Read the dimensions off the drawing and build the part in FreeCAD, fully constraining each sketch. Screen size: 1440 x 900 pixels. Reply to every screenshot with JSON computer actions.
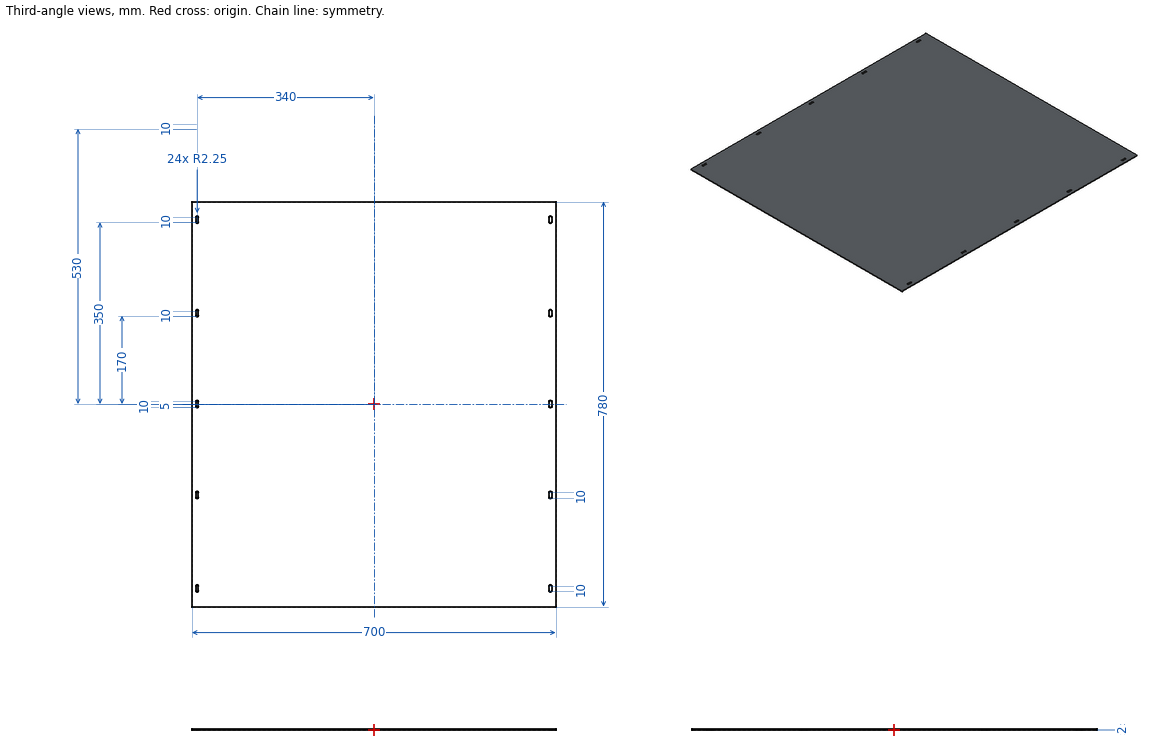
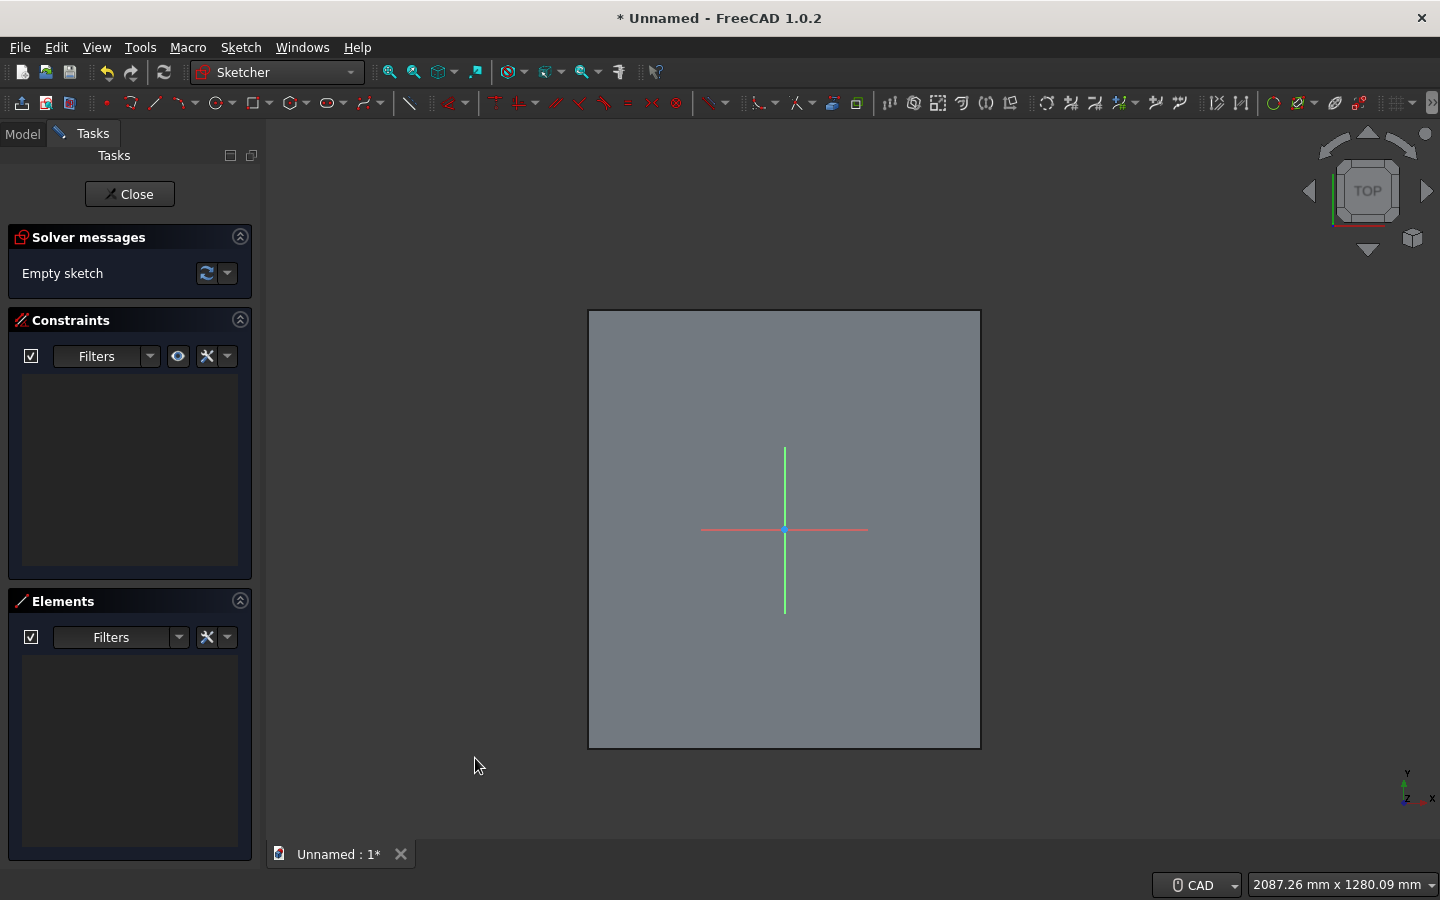
{"action": "key", "text": "g s"}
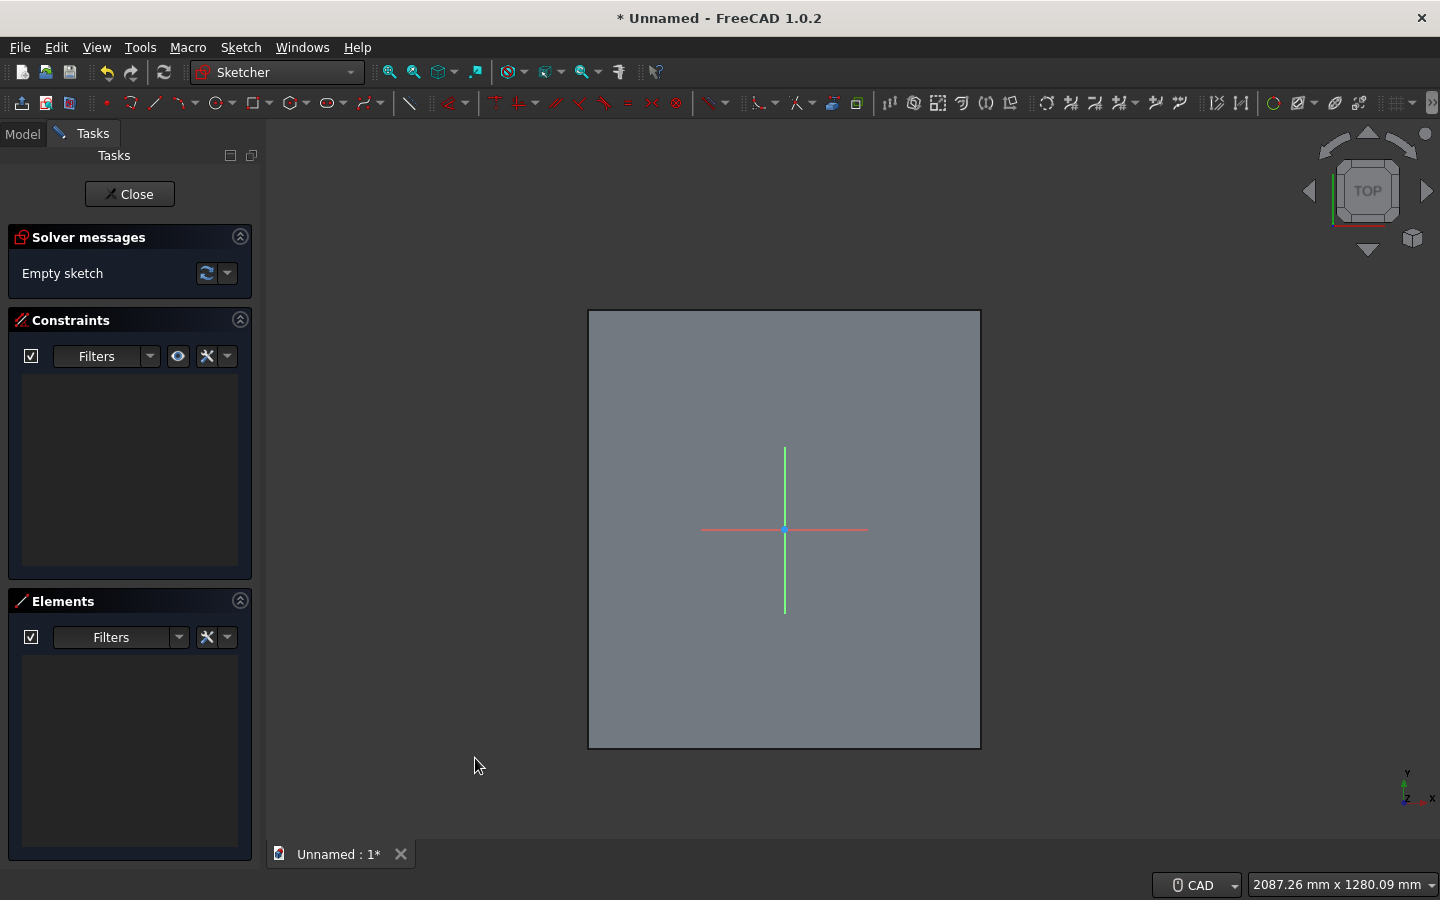
{"action": "scroll", "coordinate": [593, 333], "scroll_direction": "up", "scroll_amount": 15}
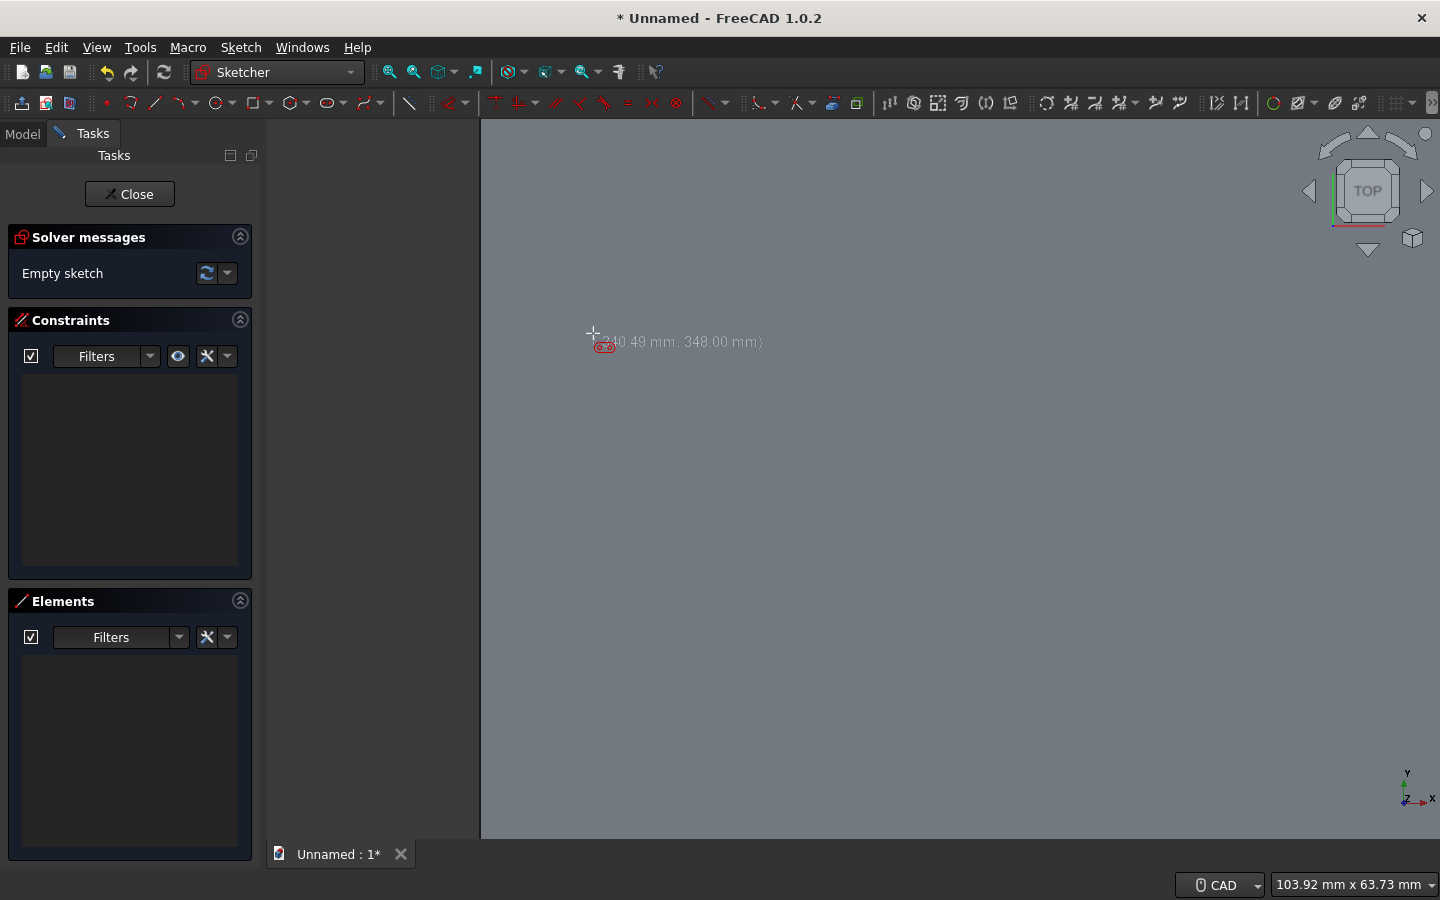
{"action": "scroll", "coordinate": [593, 333], "scroll_direction": "down", "scroll_amount": 15}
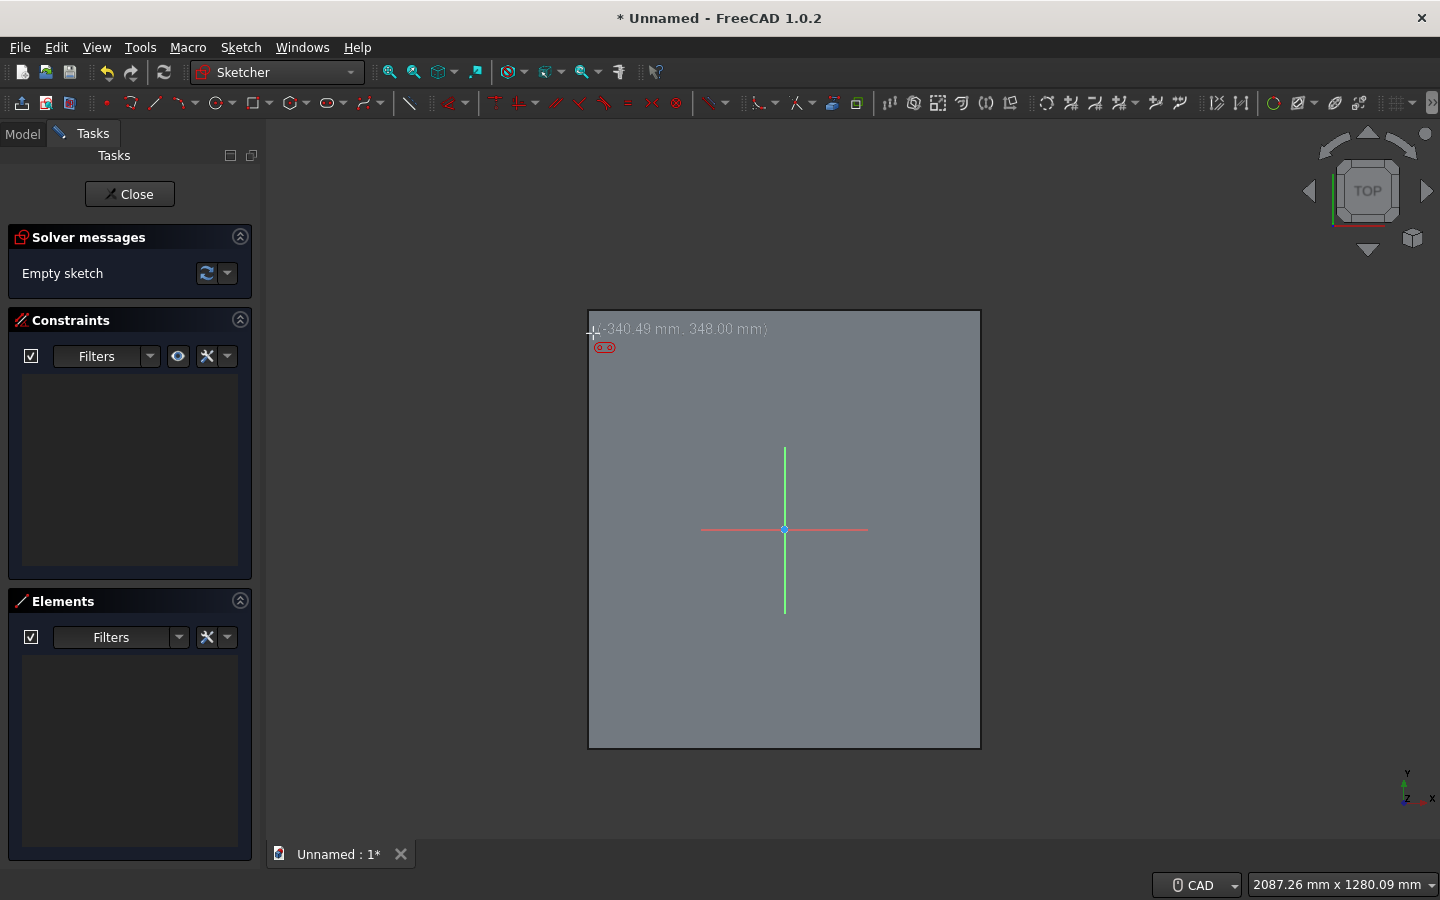
{"action": "left_click", "coordinate": [593, 333]}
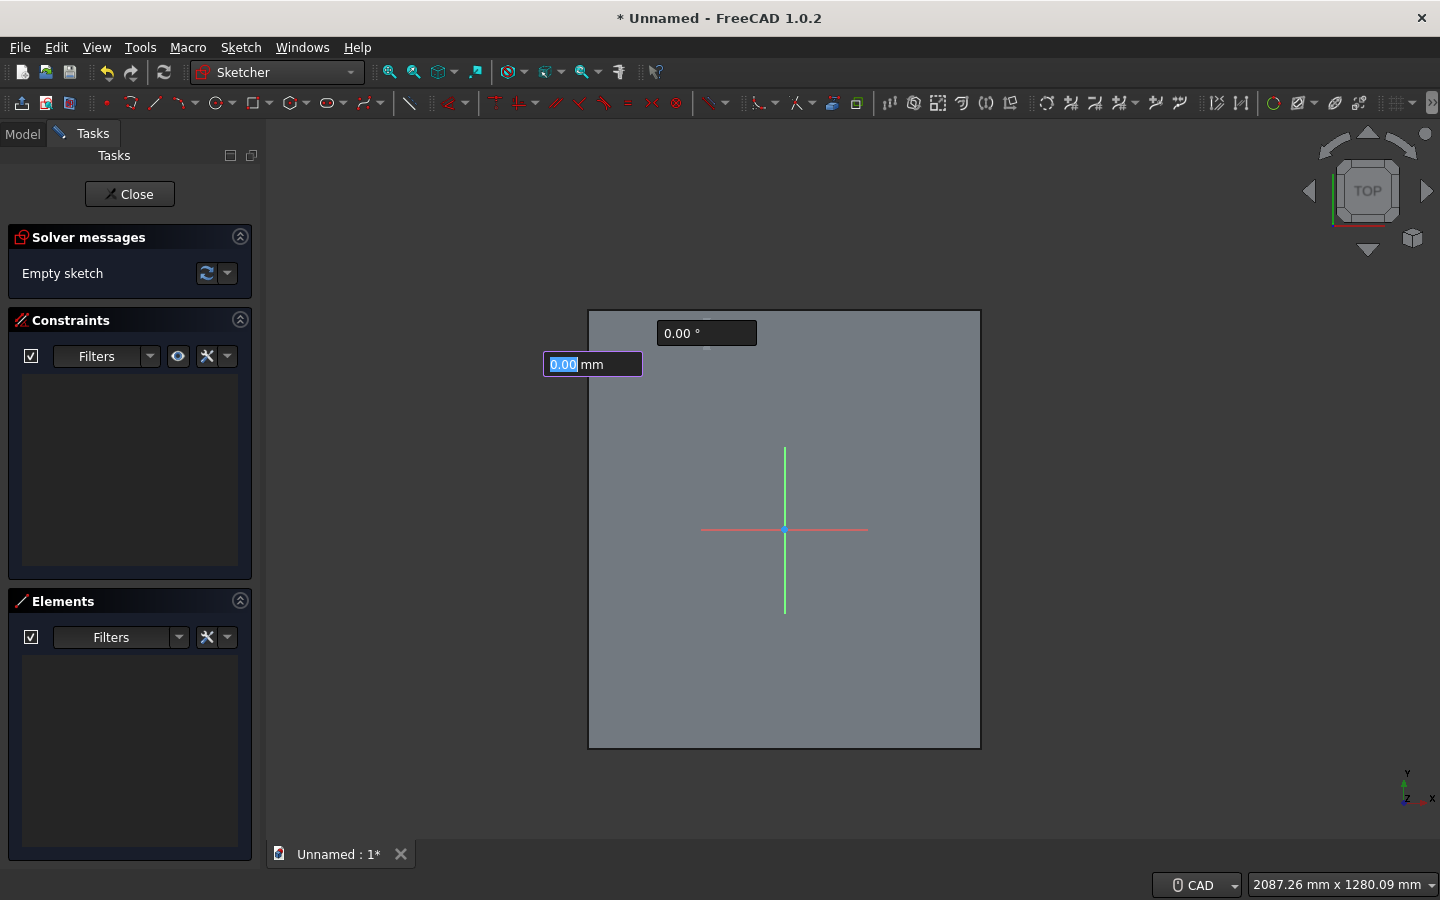
{"action": "scroll", "coordinate": [593, 327], "scroll_direction": "up", "scroll_amount": 6}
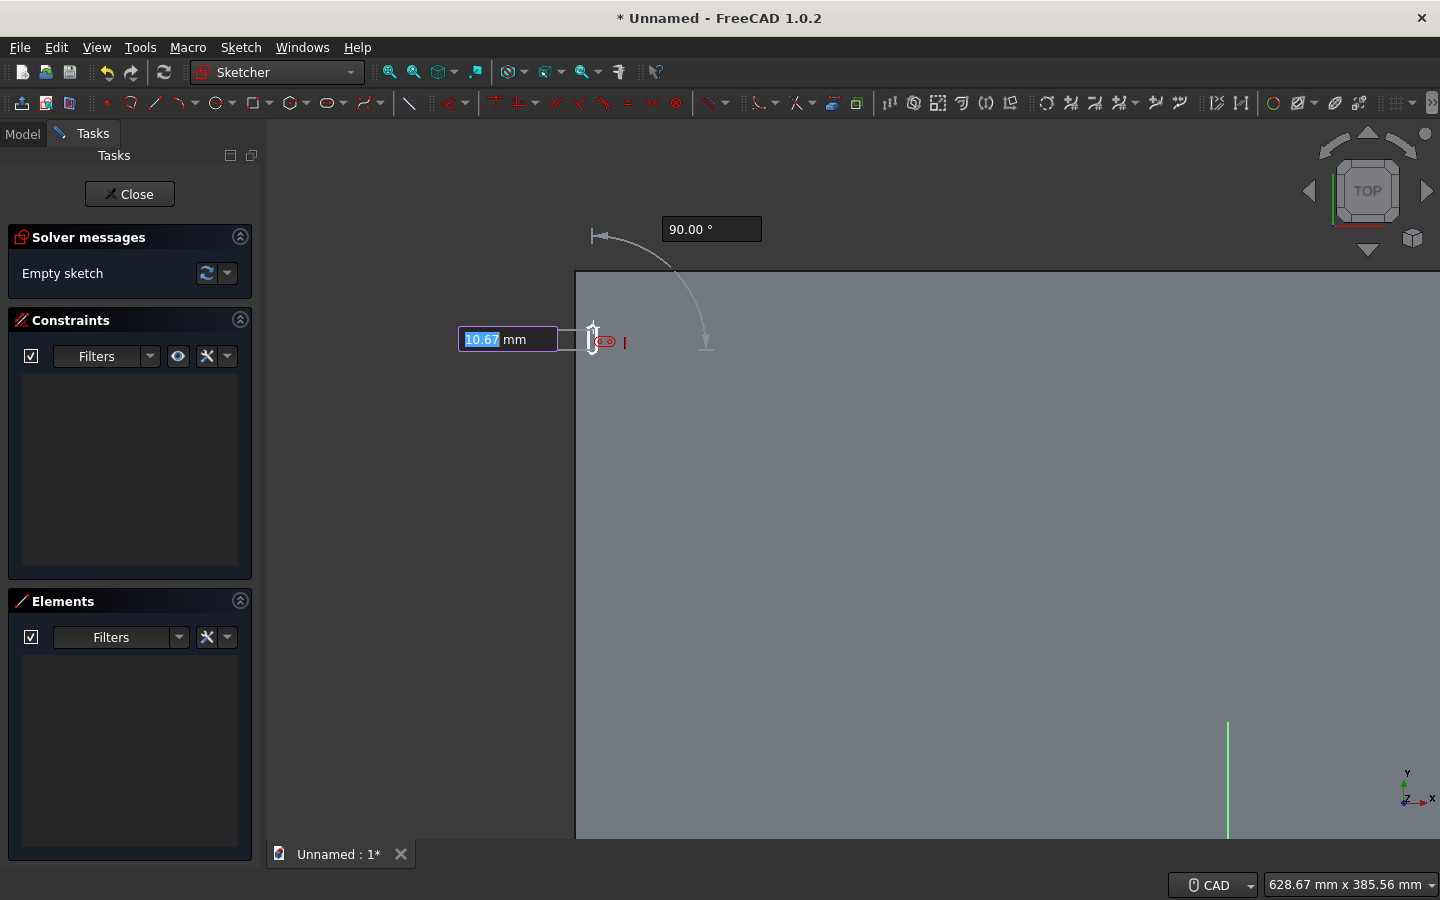
{"action": "left_click", "coordinate": [592, 327]}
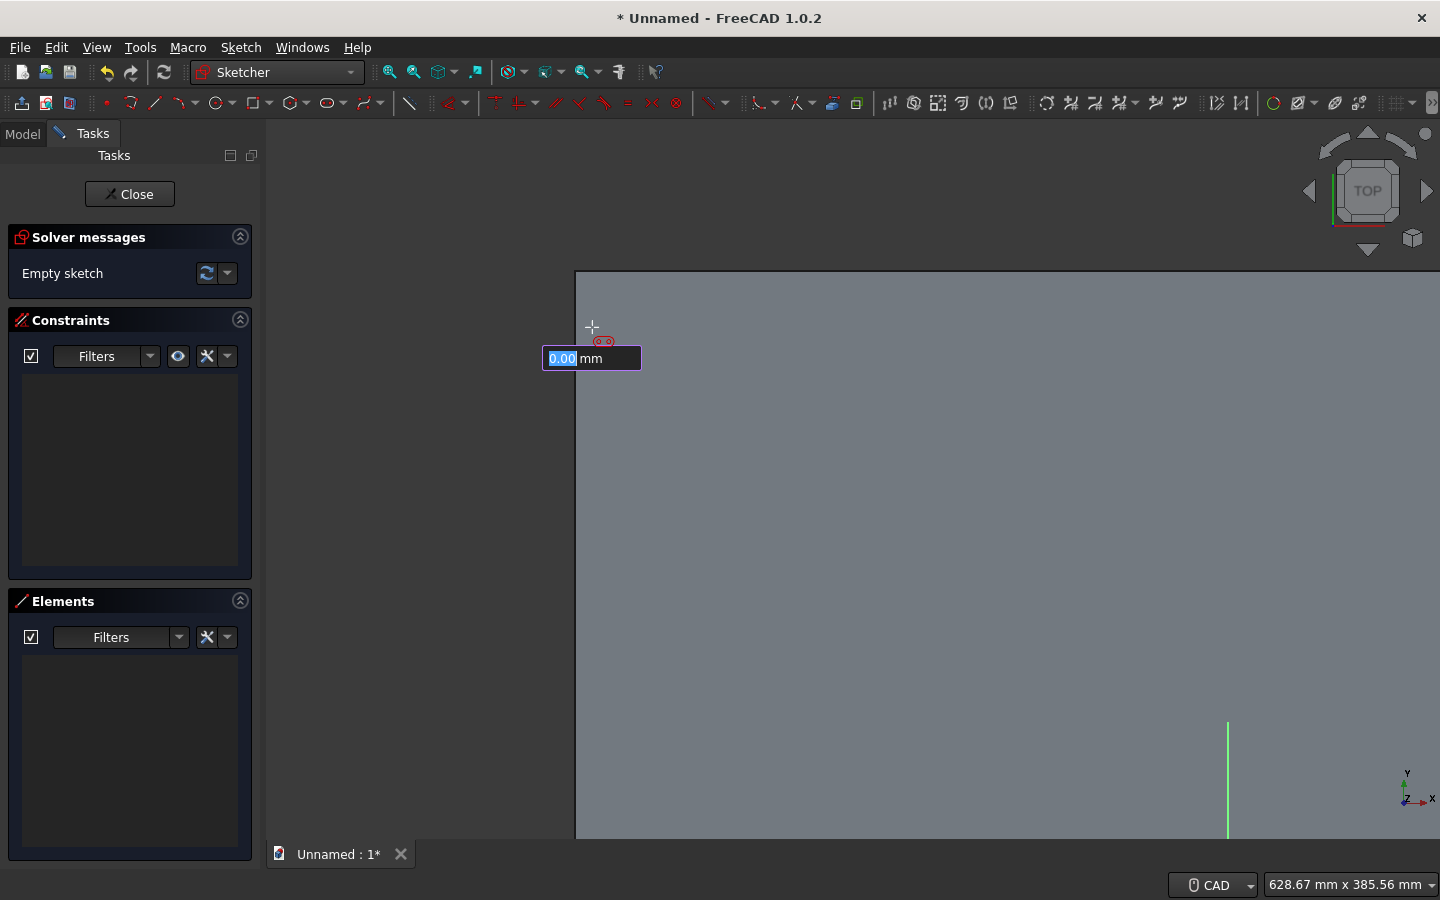
{"action": "scroll", "coordinate": [597, 336], "scroll_direction": "up", "scroll_amount": 7}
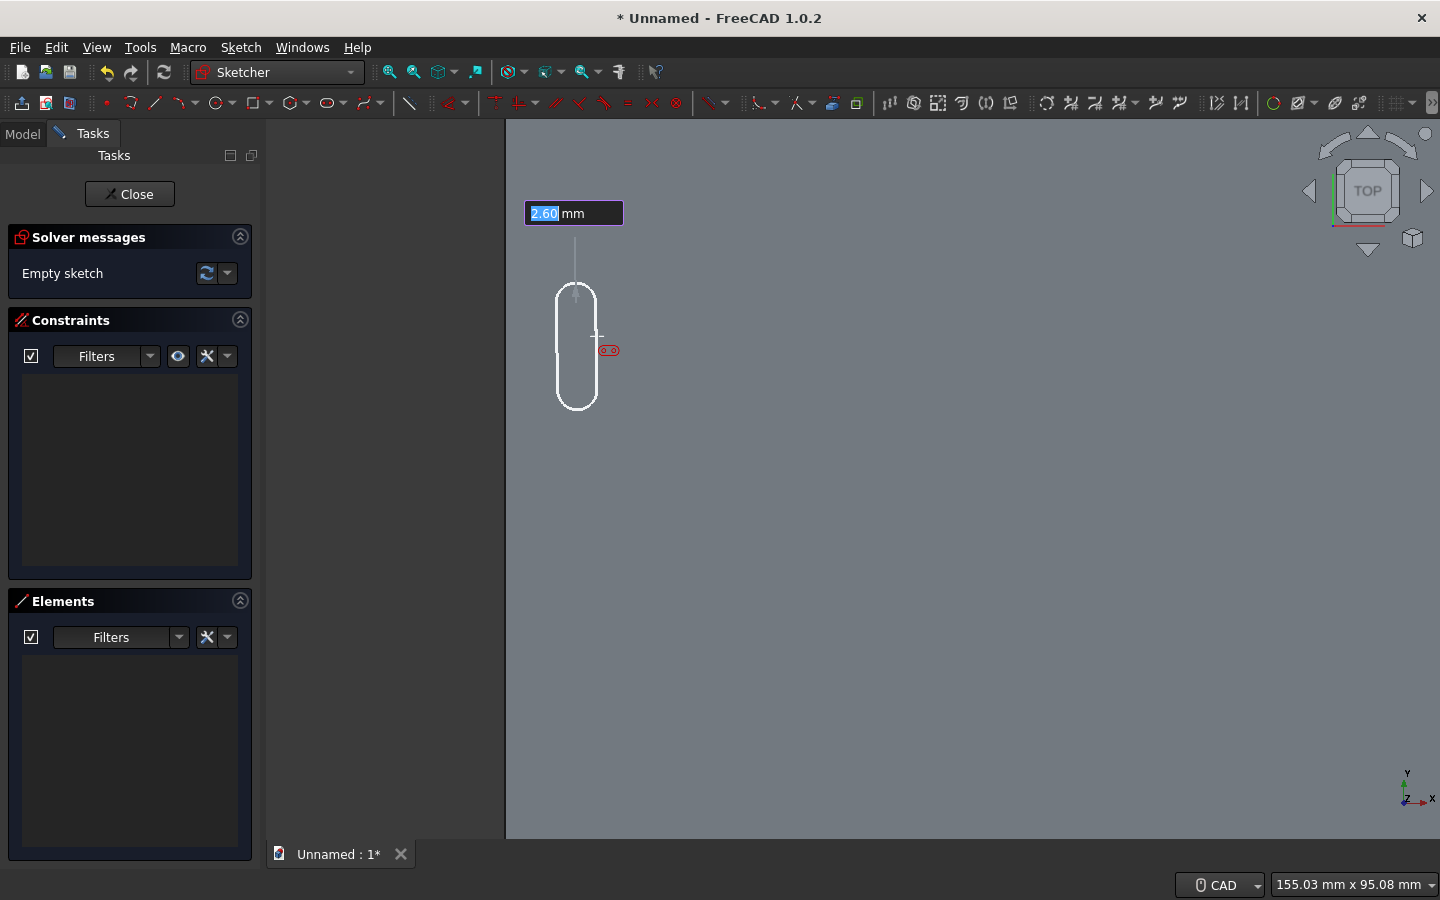
{"action": "left_click", "coordinate": [598, 337]}